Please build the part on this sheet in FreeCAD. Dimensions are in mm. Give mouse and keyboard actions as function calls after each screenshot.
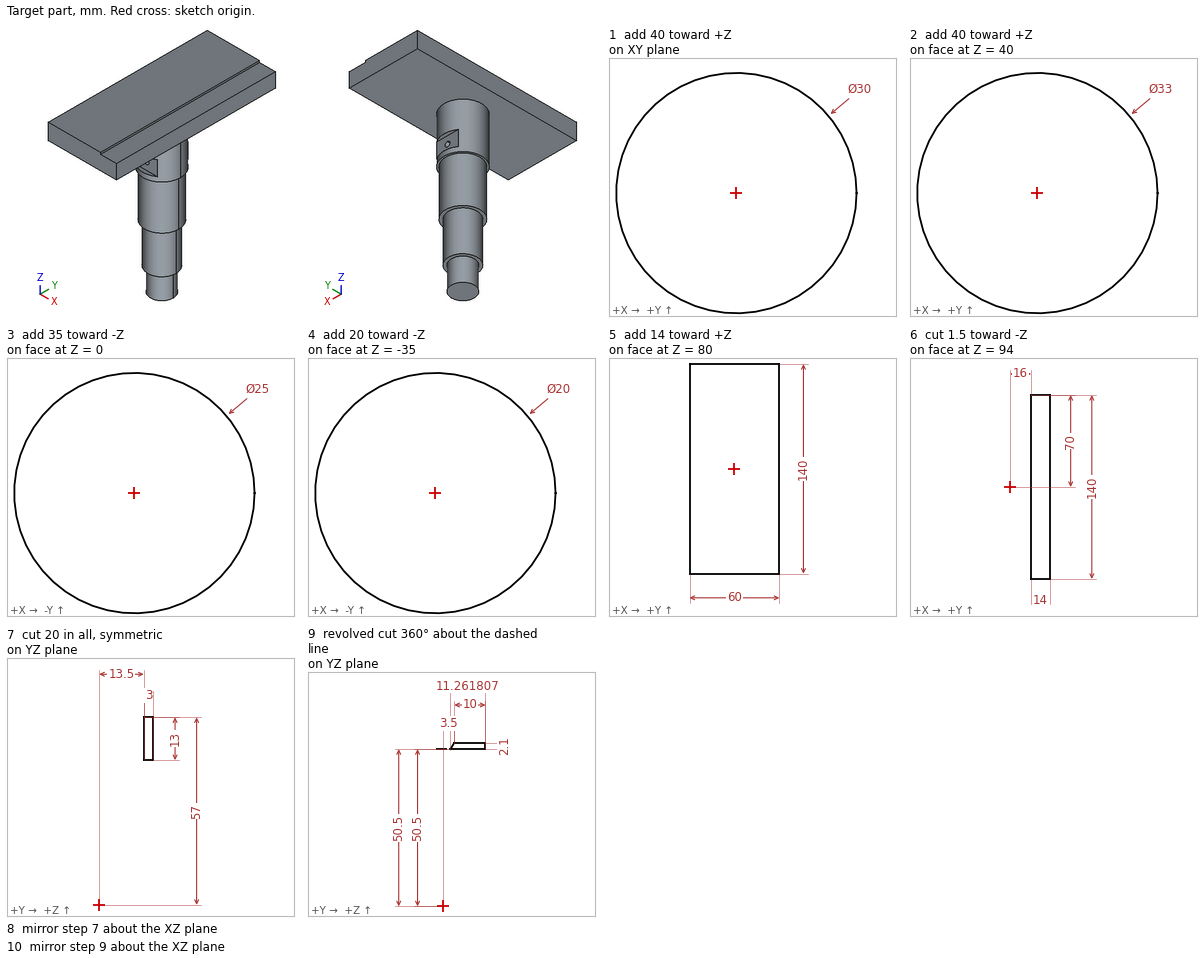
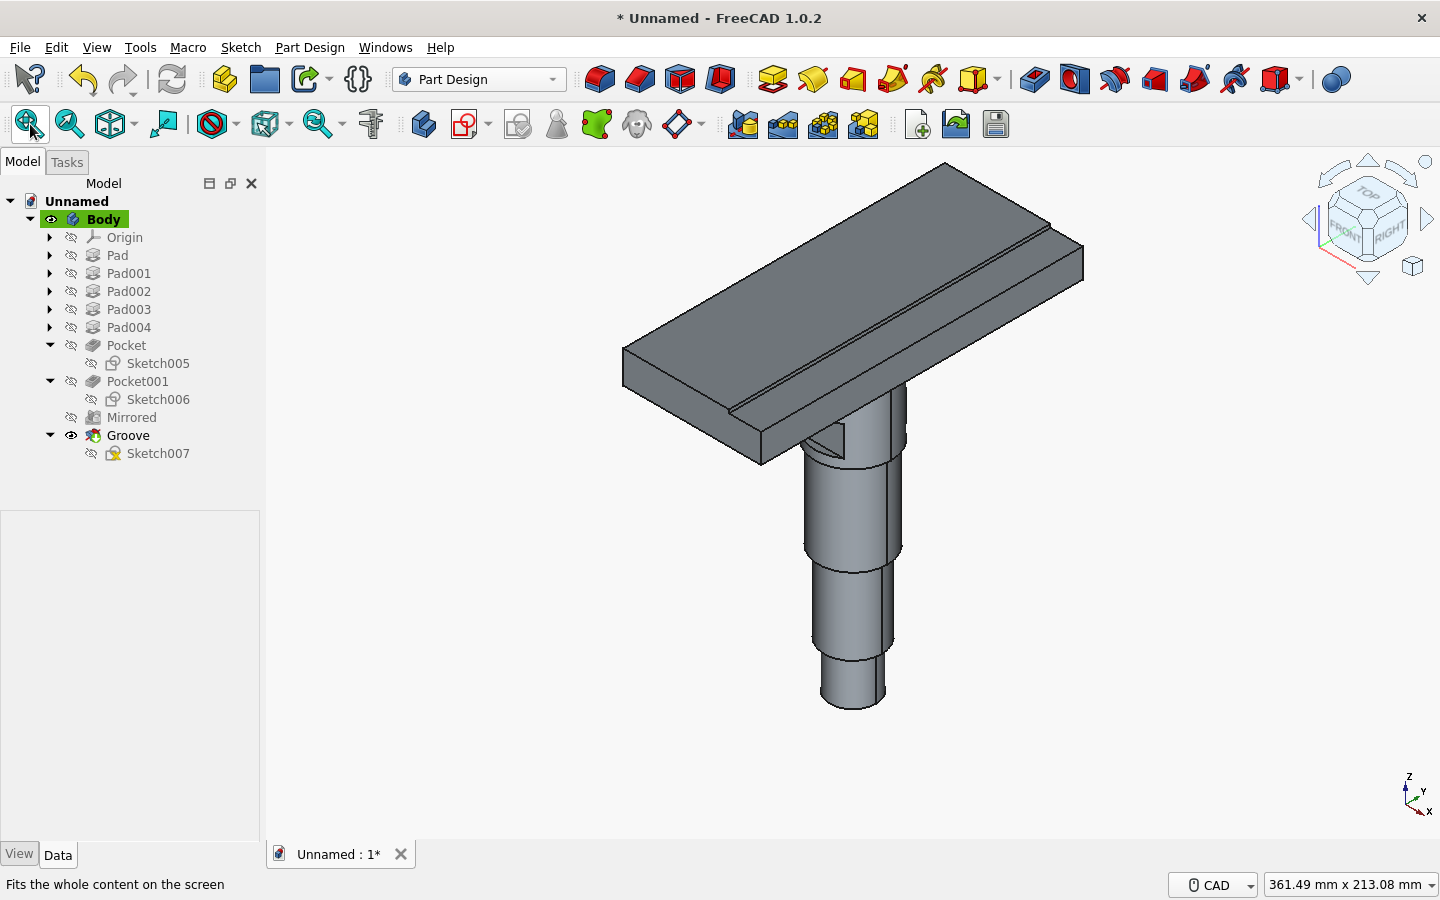
click(116, 435)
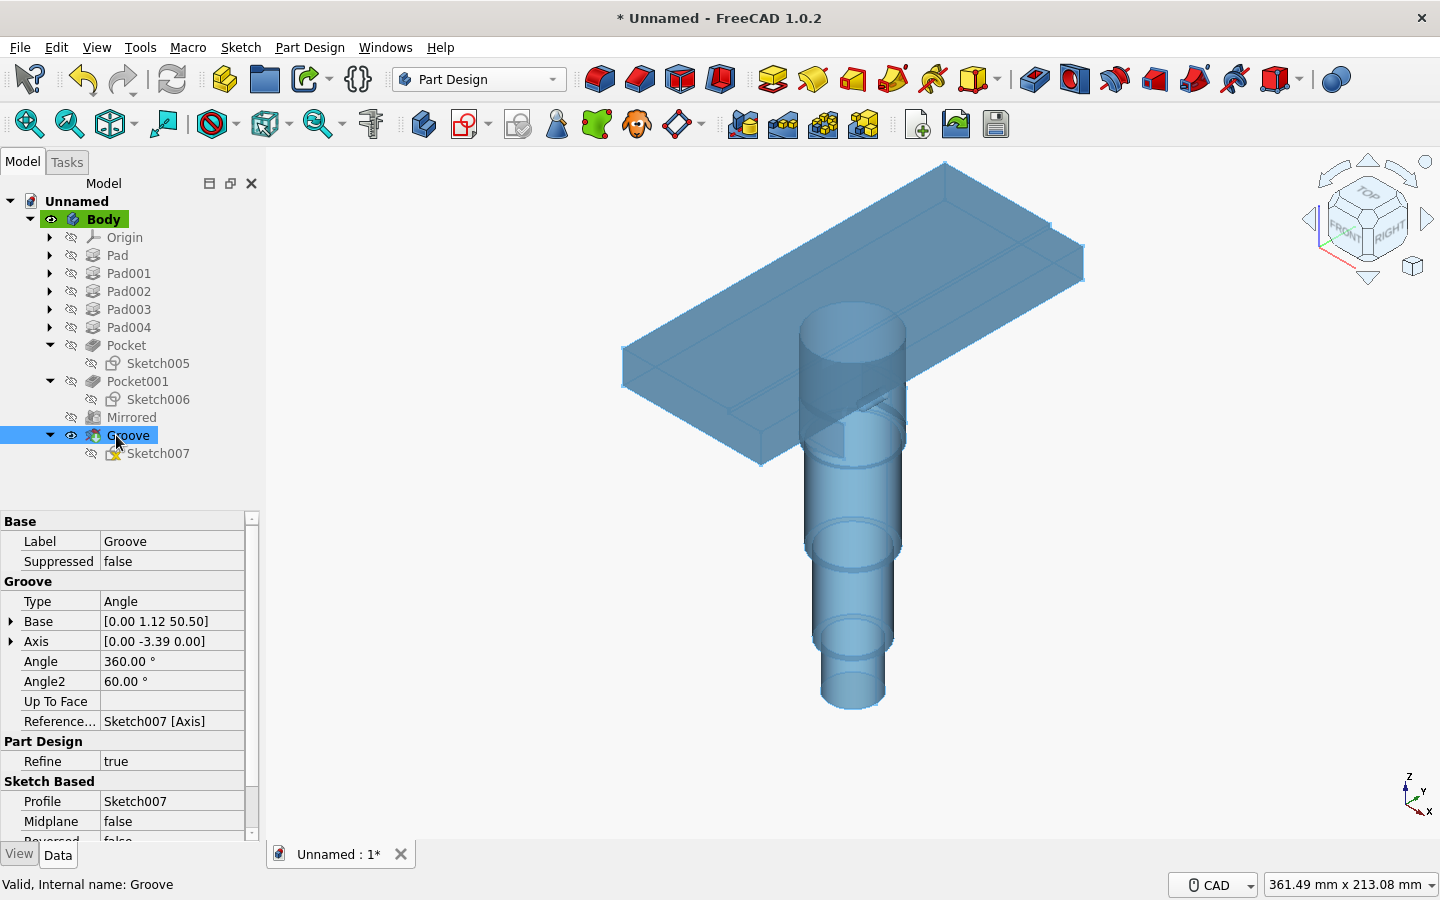
click(744, 124)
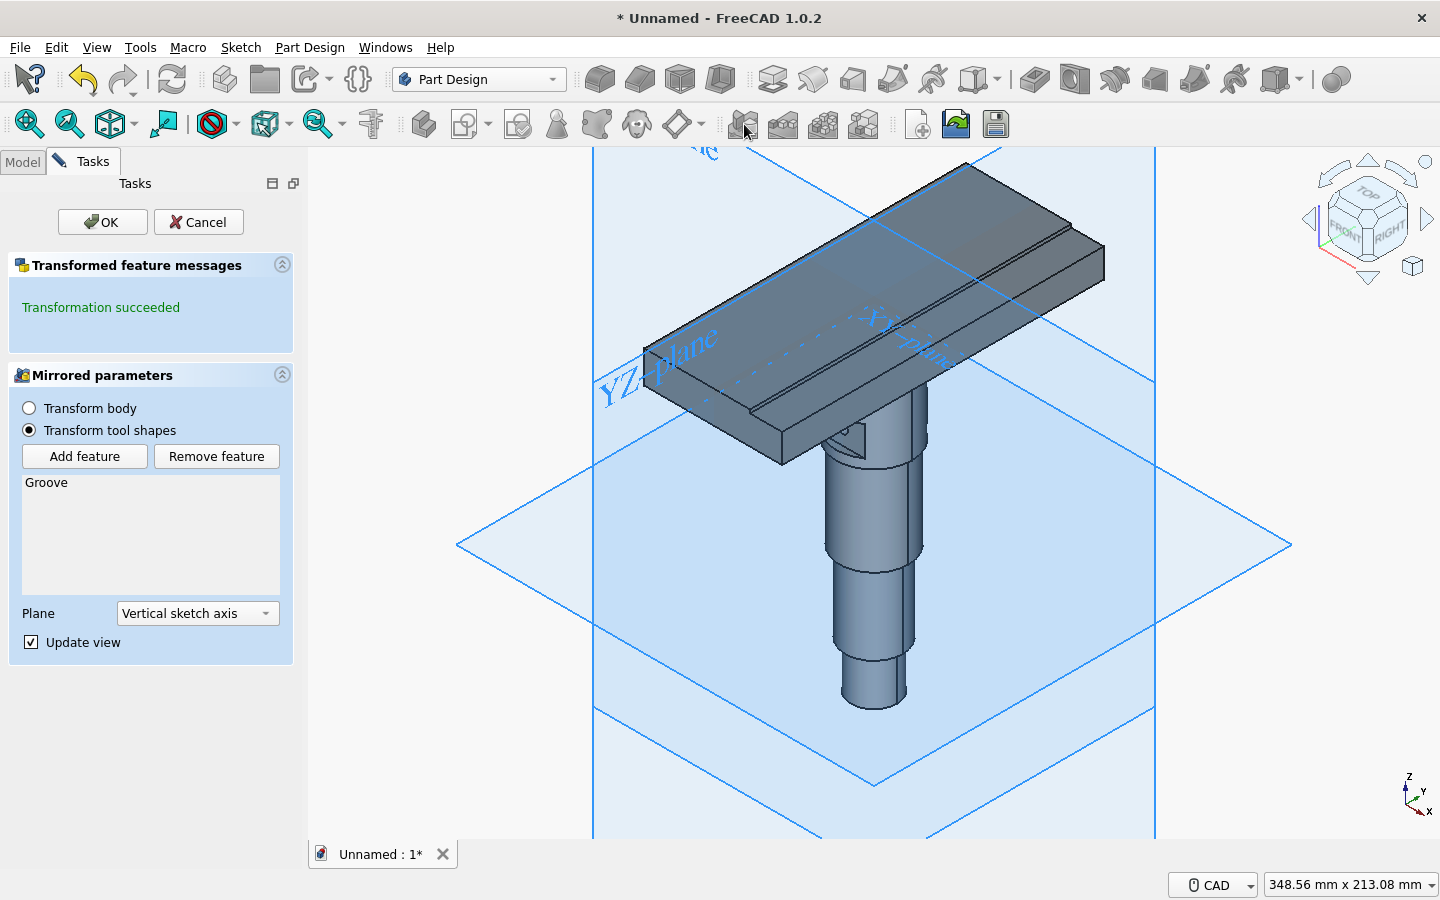
click(198, 614)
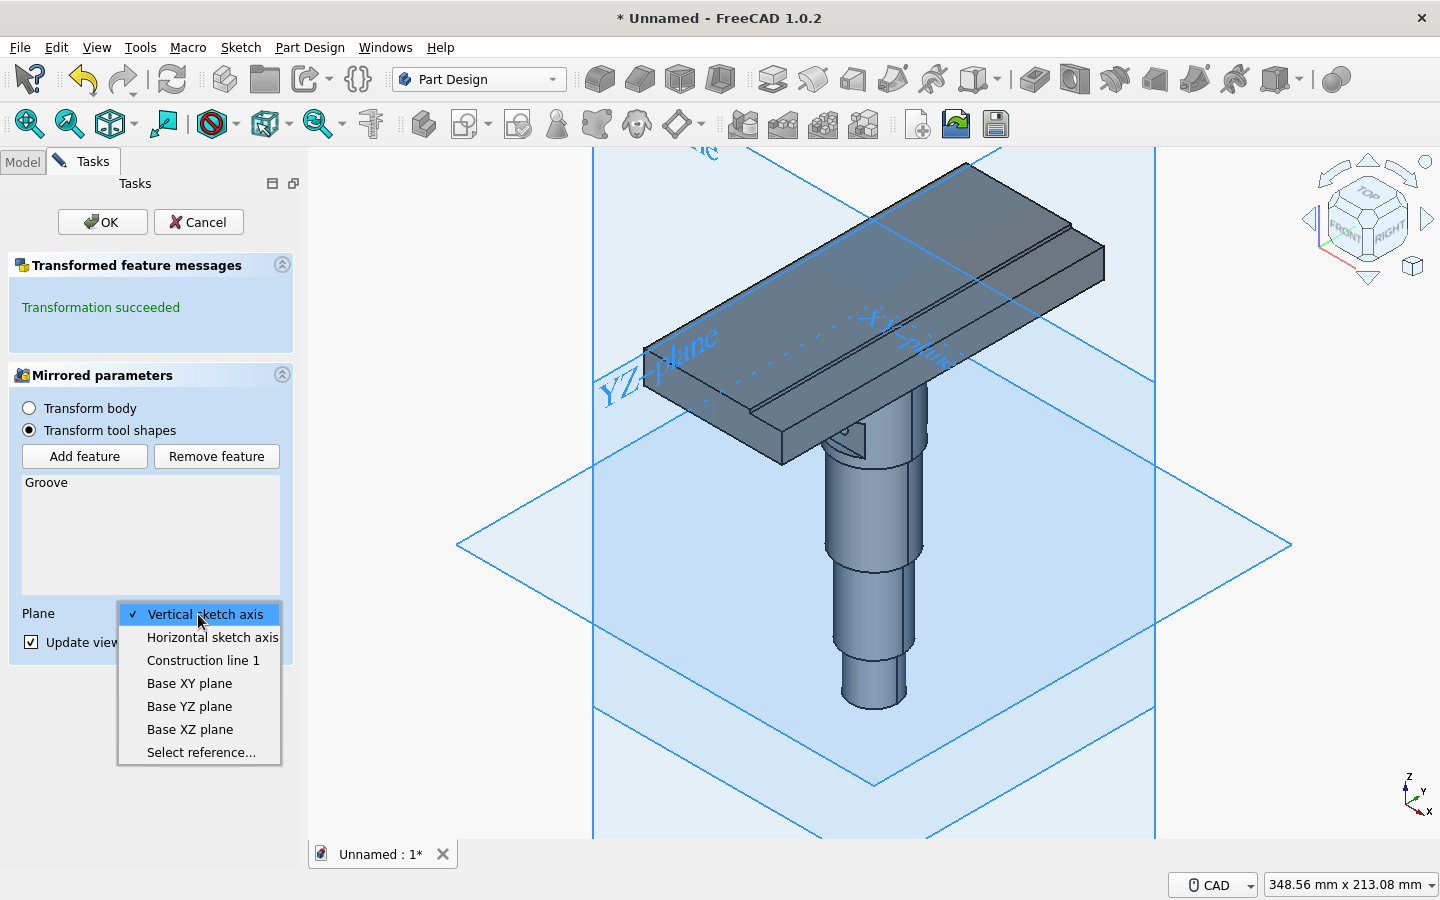
click(198, 730)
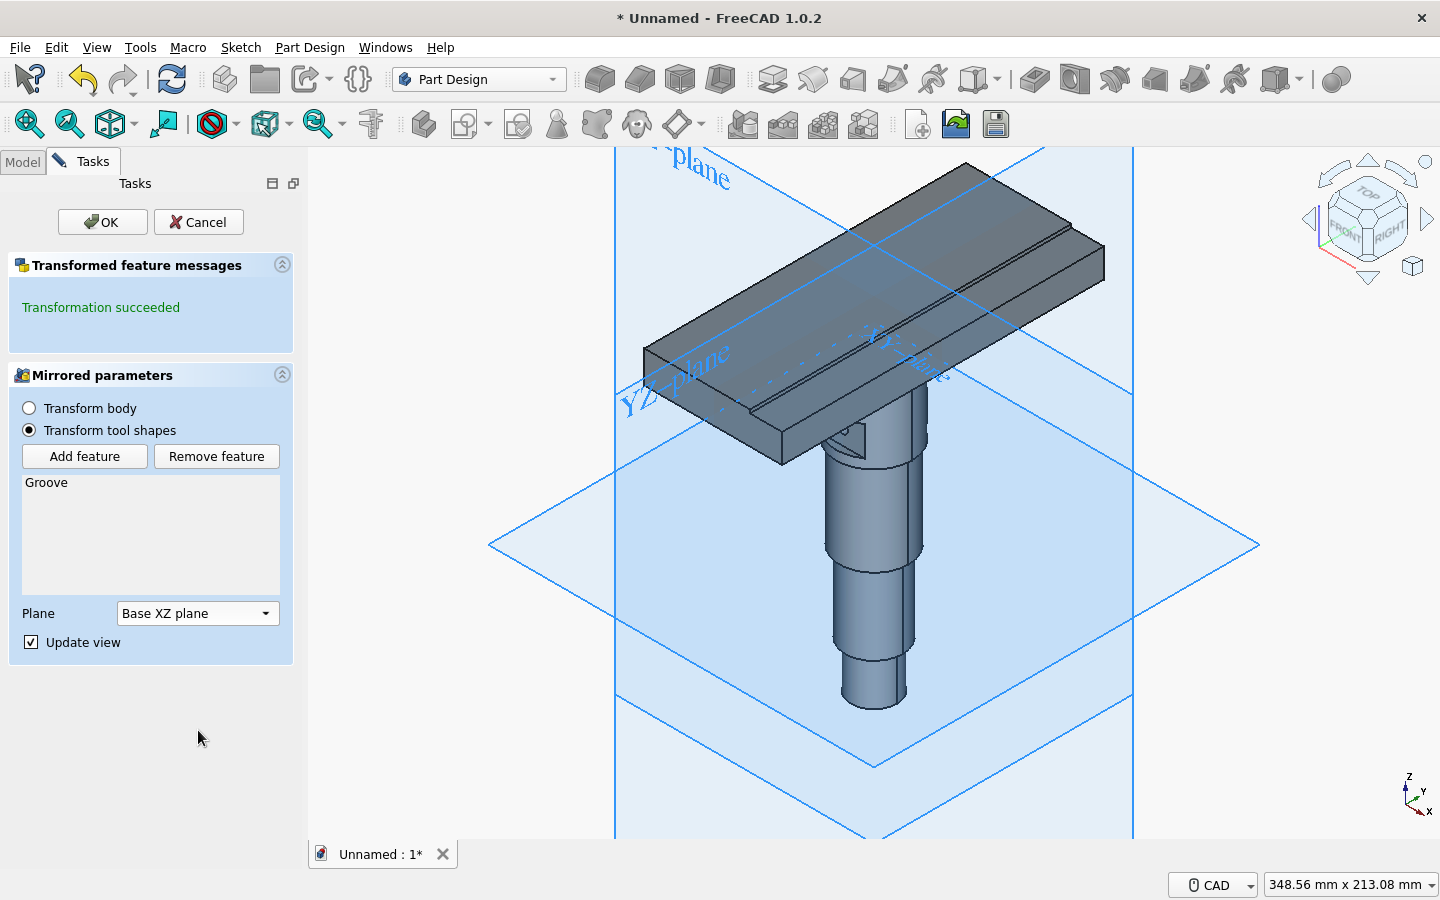
click(103, 222)